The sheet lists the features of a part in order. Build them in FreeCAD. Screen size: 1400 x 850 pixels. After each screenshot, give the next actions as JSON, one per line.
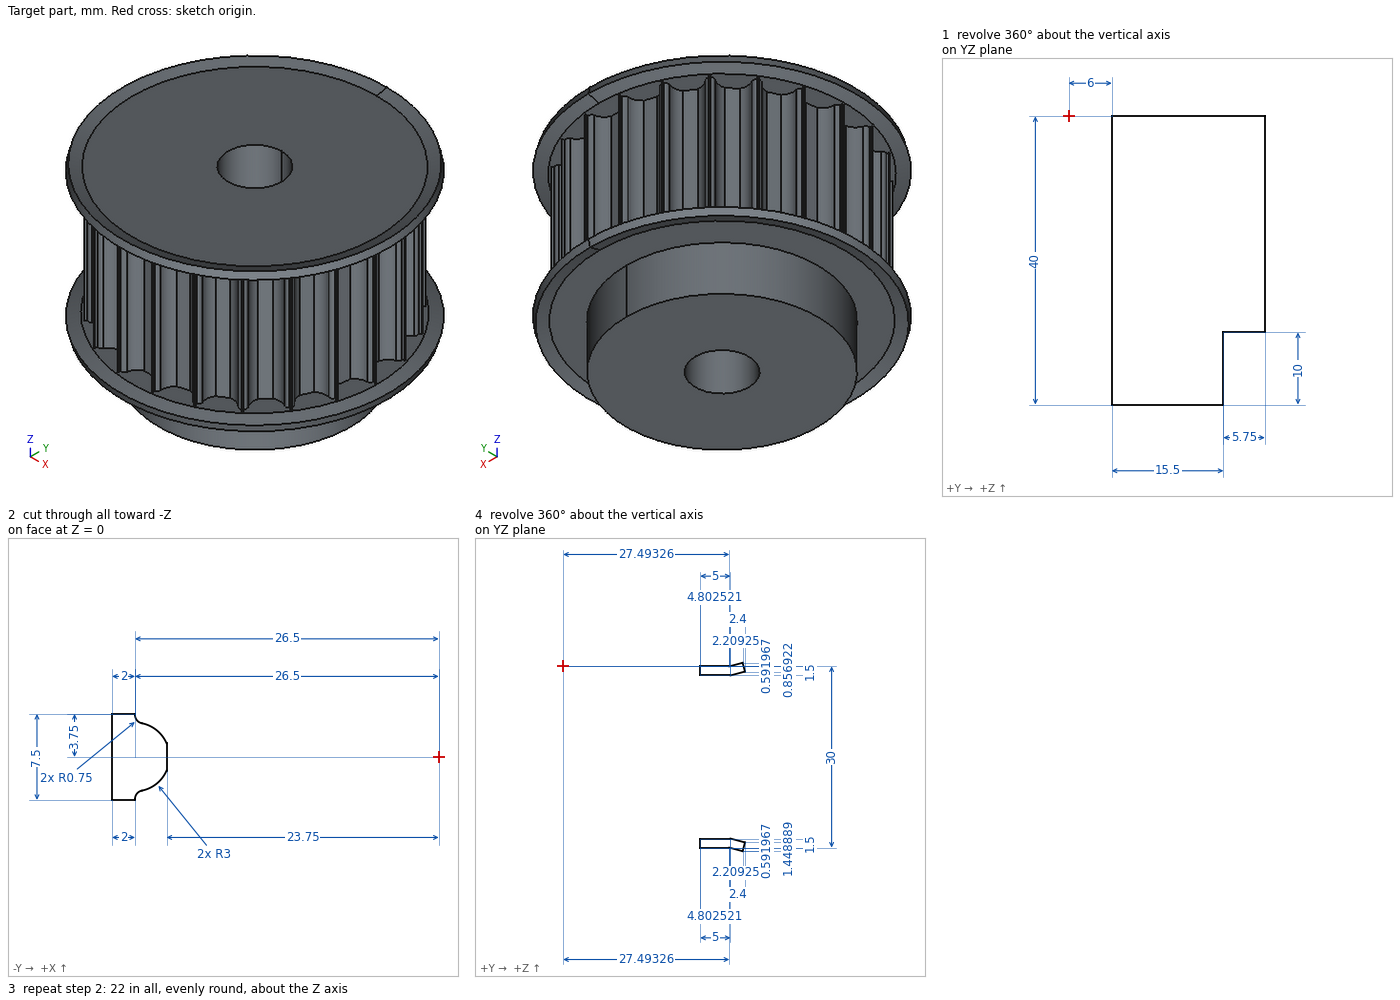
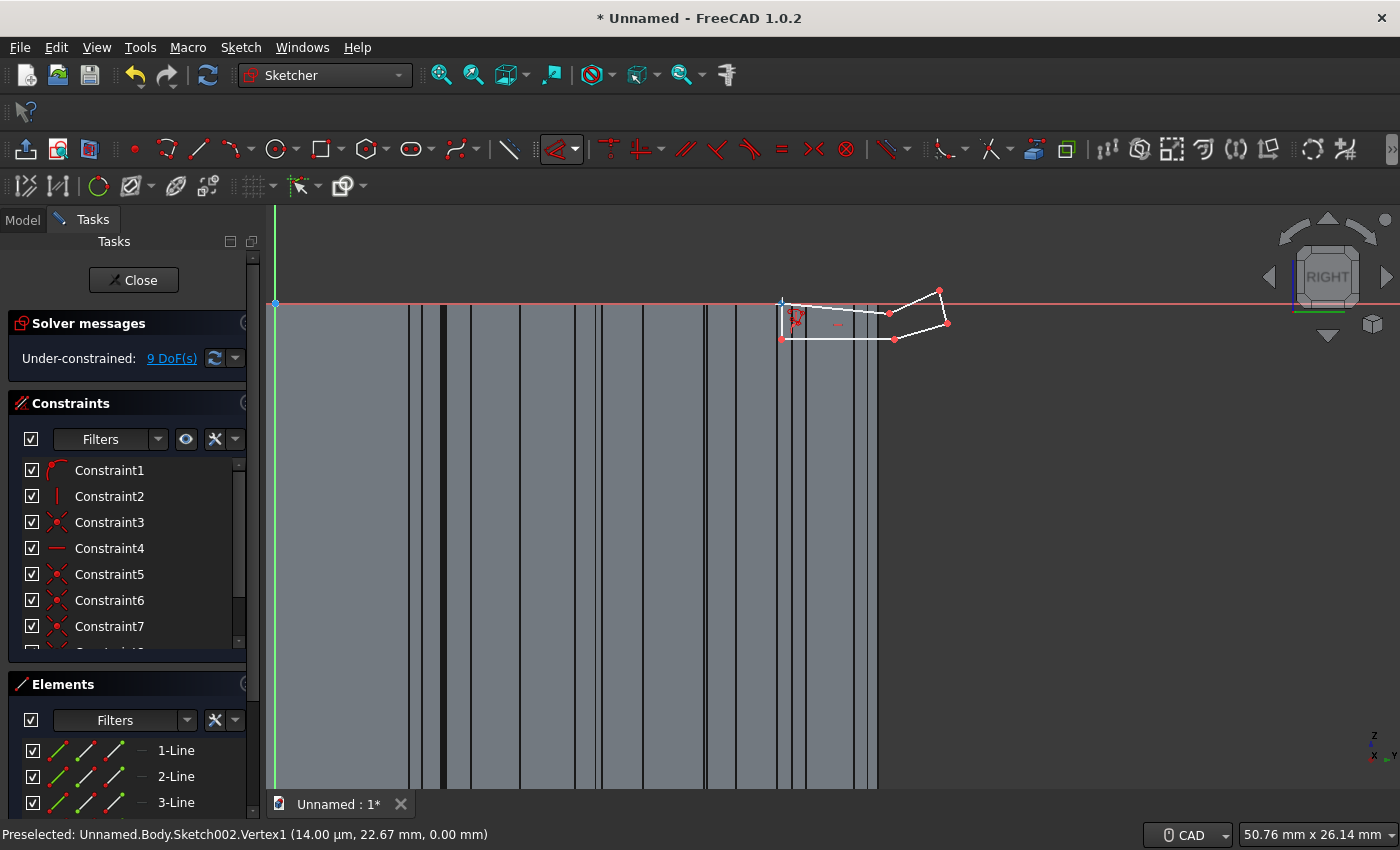
{"action": "scroll", "coordinate": [951, 325], "scroll_direction": "down", "scroll_amount": 3}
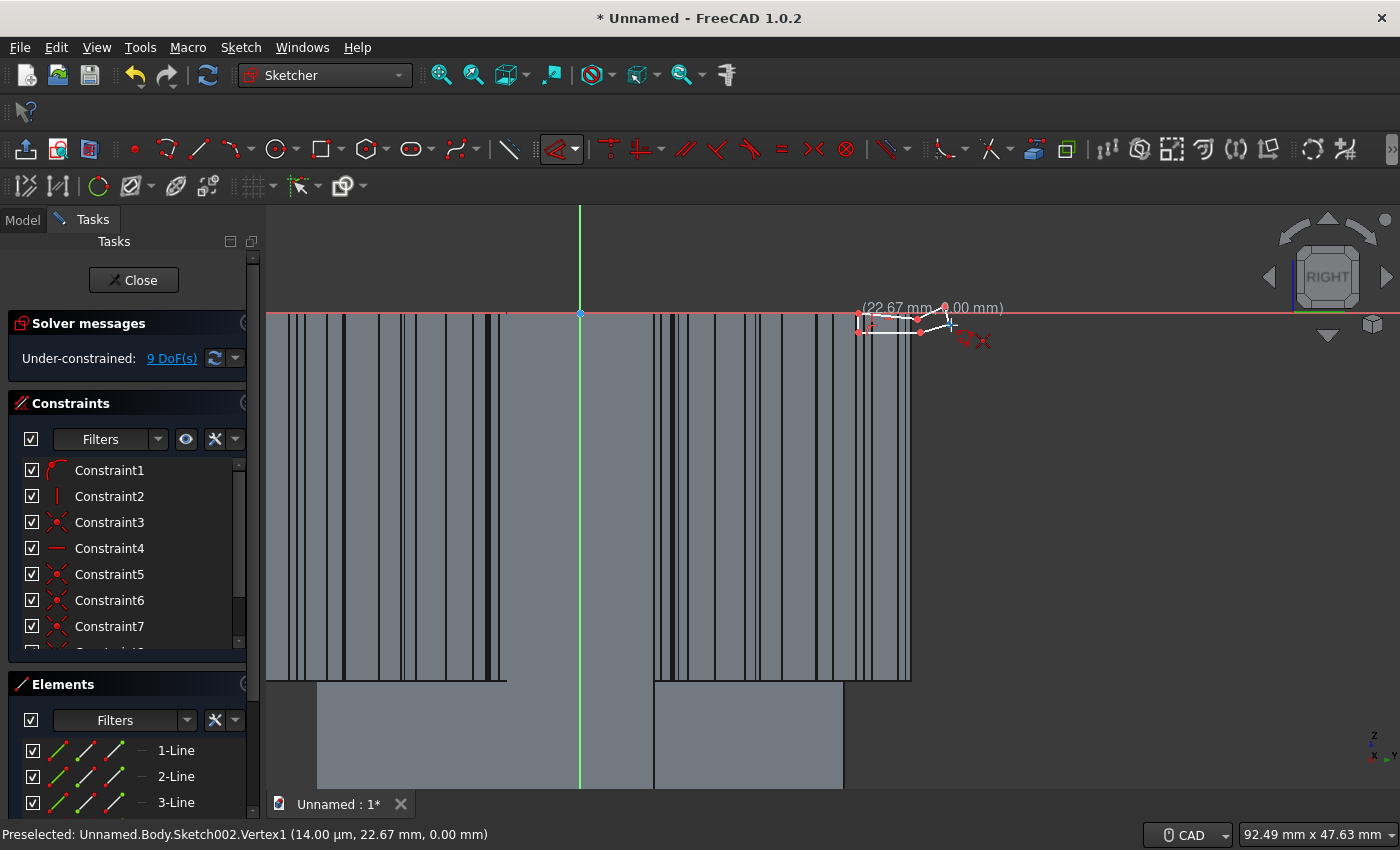
{"action": "left_click", "coordinate": [859, 663]}
{"action": "left_click", "coordinate": [859, 681]}
{"action": "left_click", "coordinate": [917, 681]}
{"action": "left_click", "coordinate": [945, 688]}
{"action": "left_click", "coordinate": [949, 671]}
{"action": "left_click", "coordinate": [920, 663]}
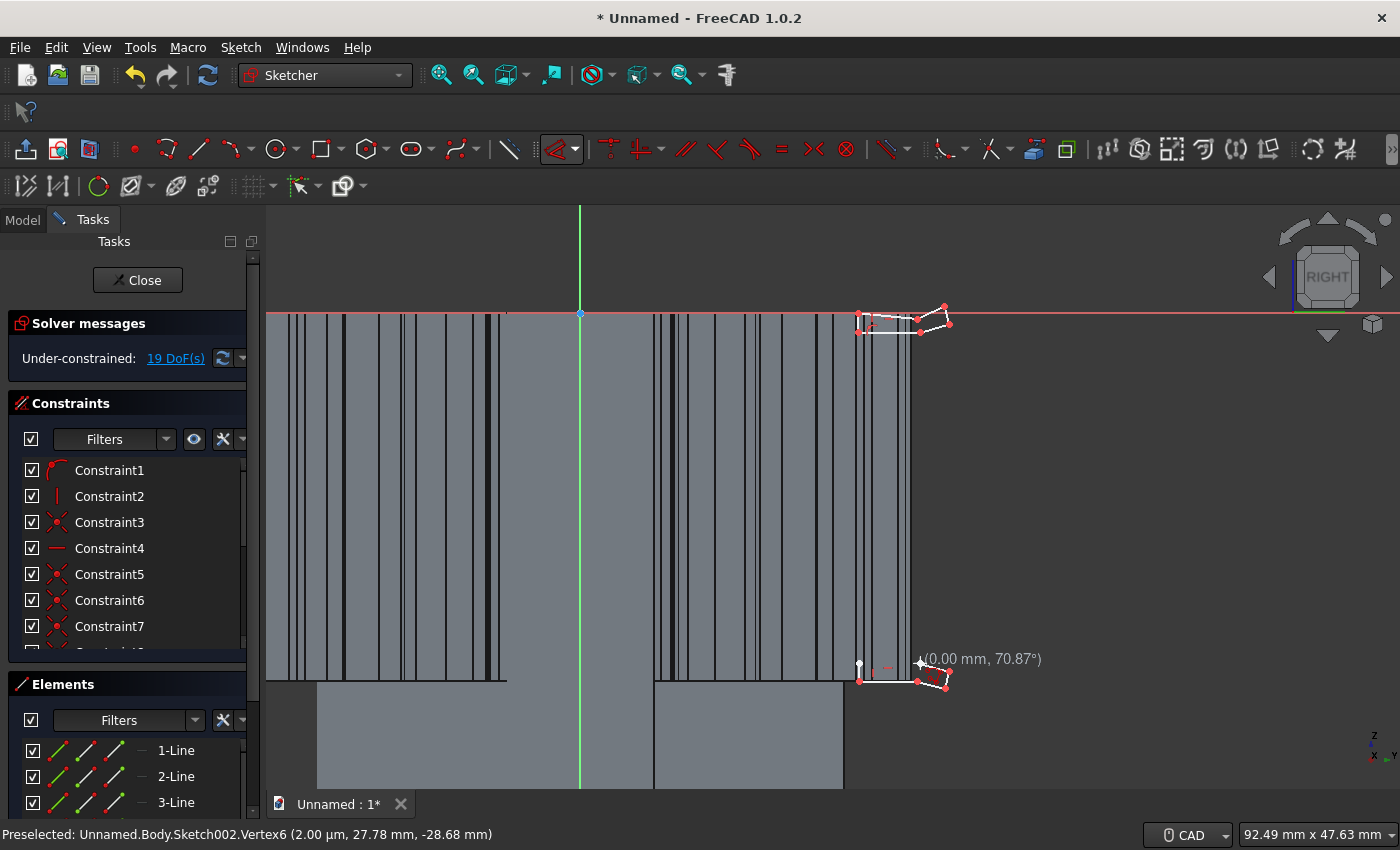
{"action": "scroll", "coordinate": [859, 663], "scroll_direction": "up", "scroll_amount": 3}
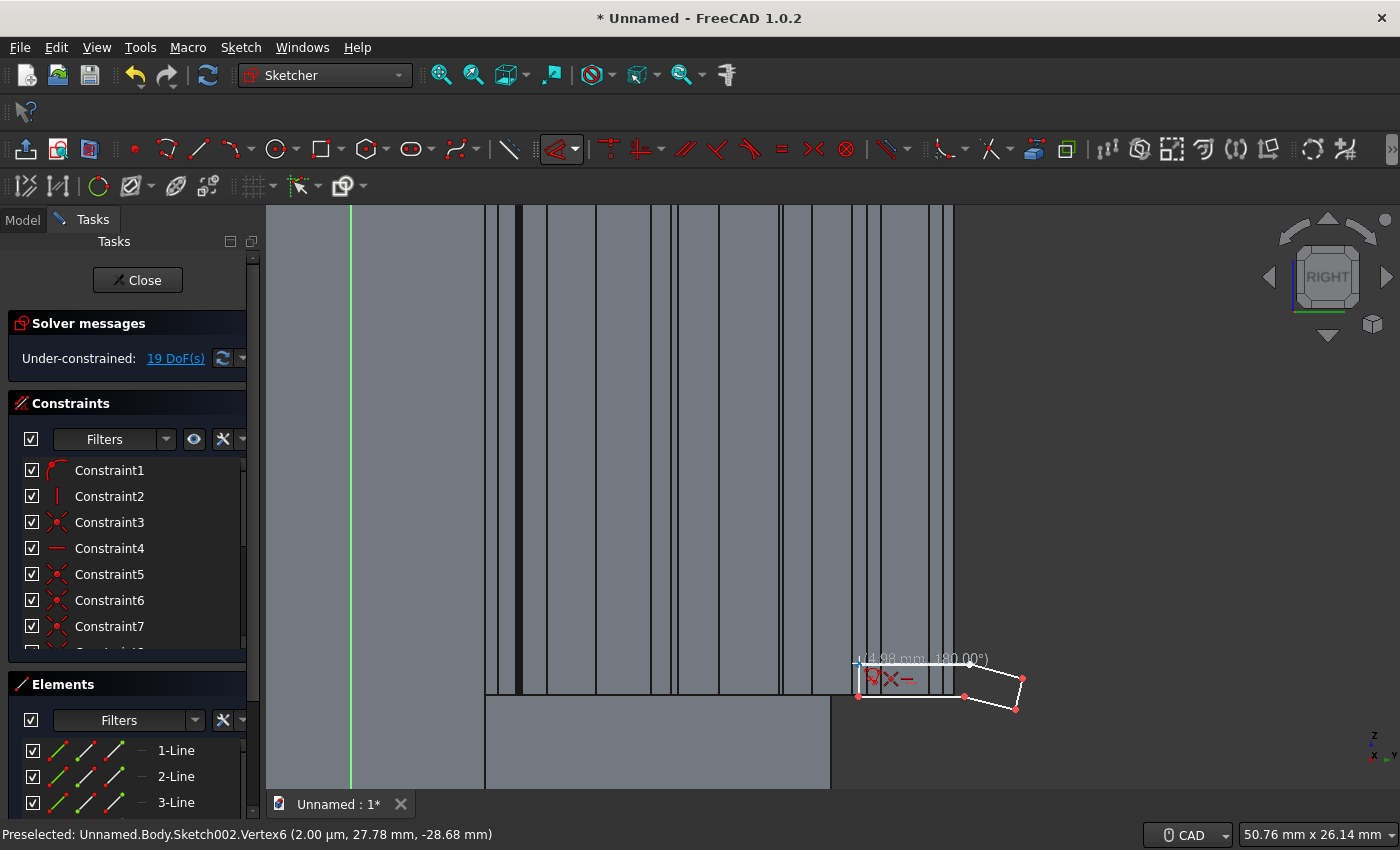
{"action": "left_click", "coordinate": [859, 664]}
{"action": "key", "text": "Escape"}
{"action": "key", "text": "Escape"}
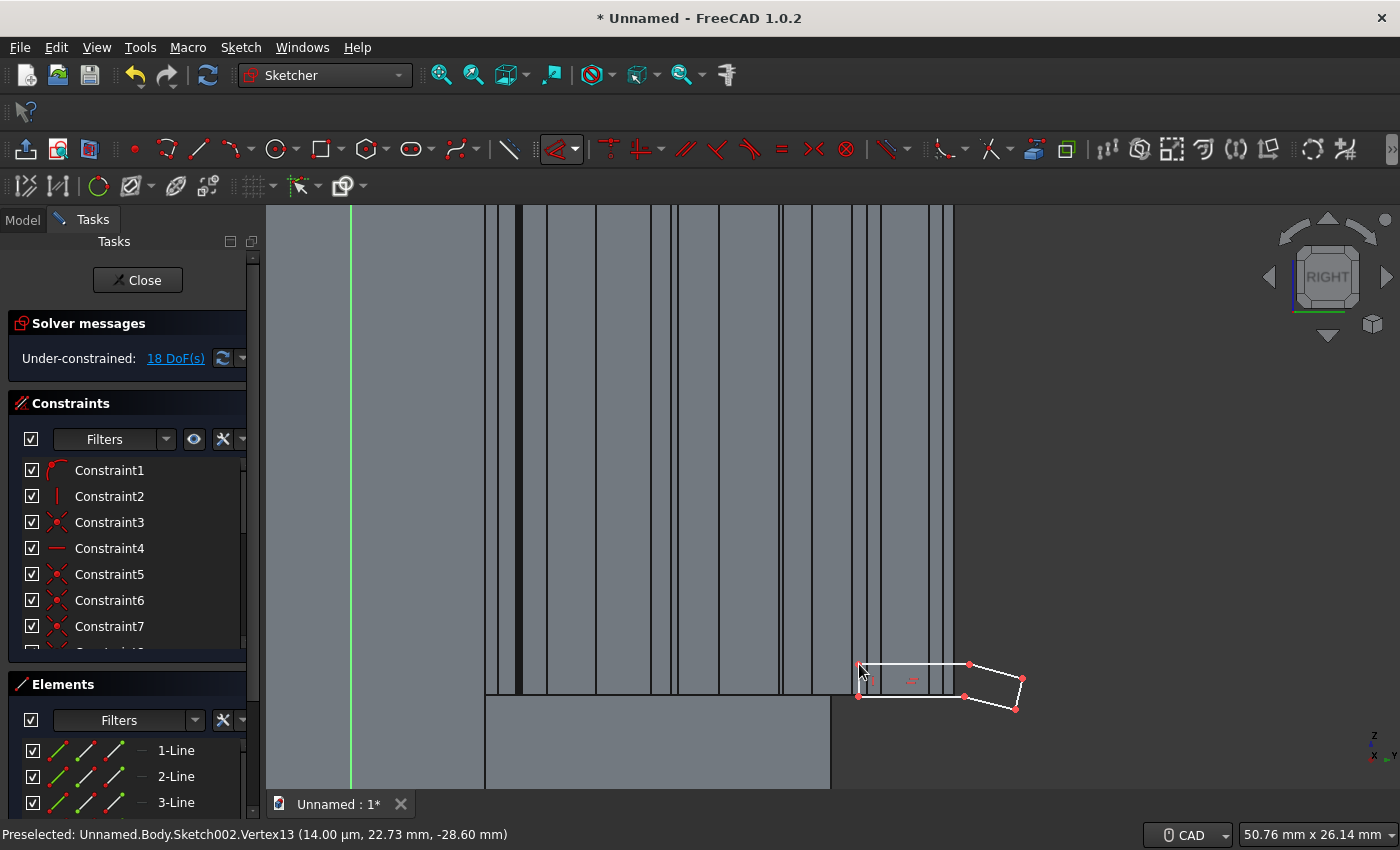
{"action": "scroll", "coordinate": [859, 663], "scroll_direction": "down", "scroll_amount": 3}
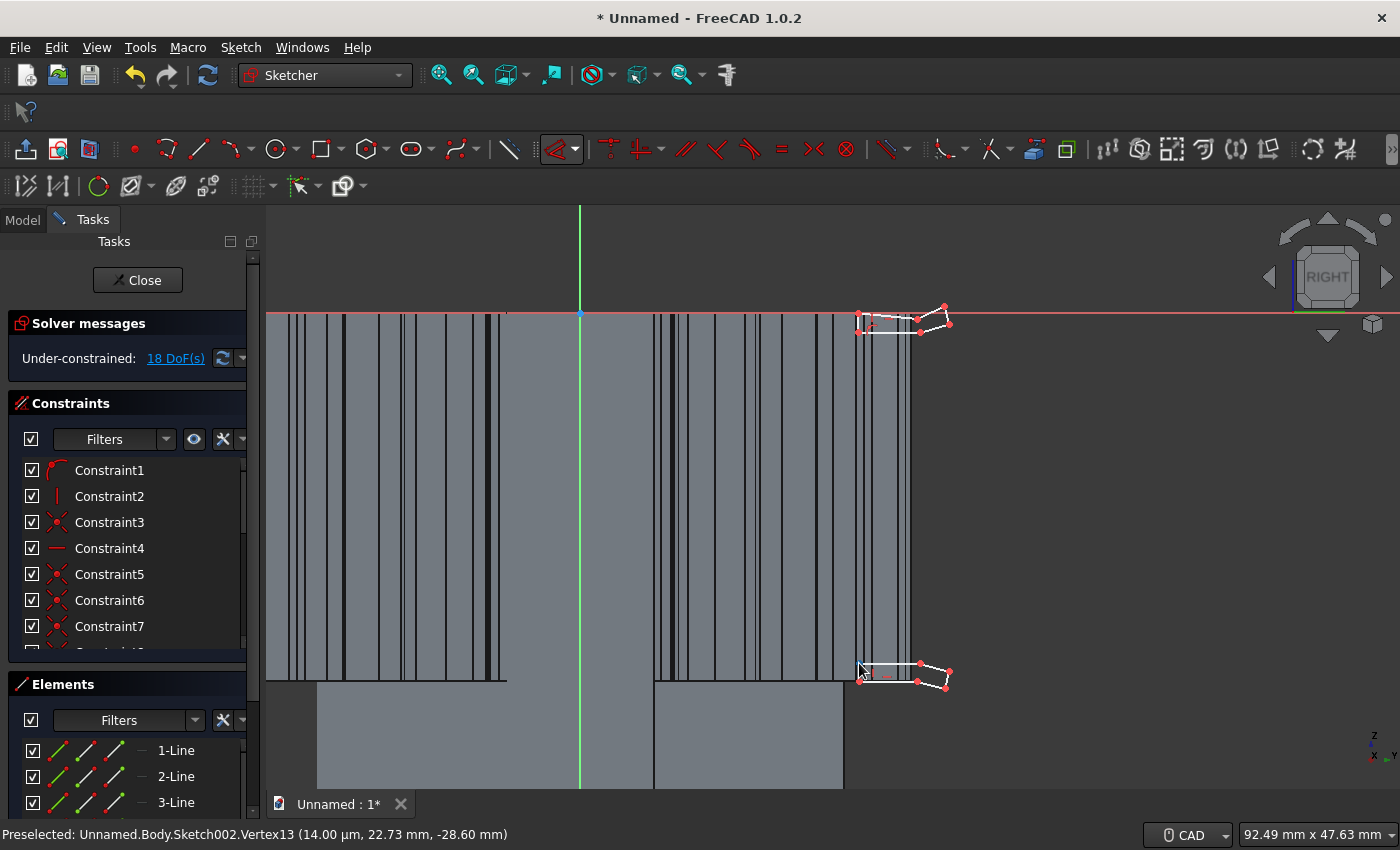
{"action": "left_click", "coordinate": [905, 318]}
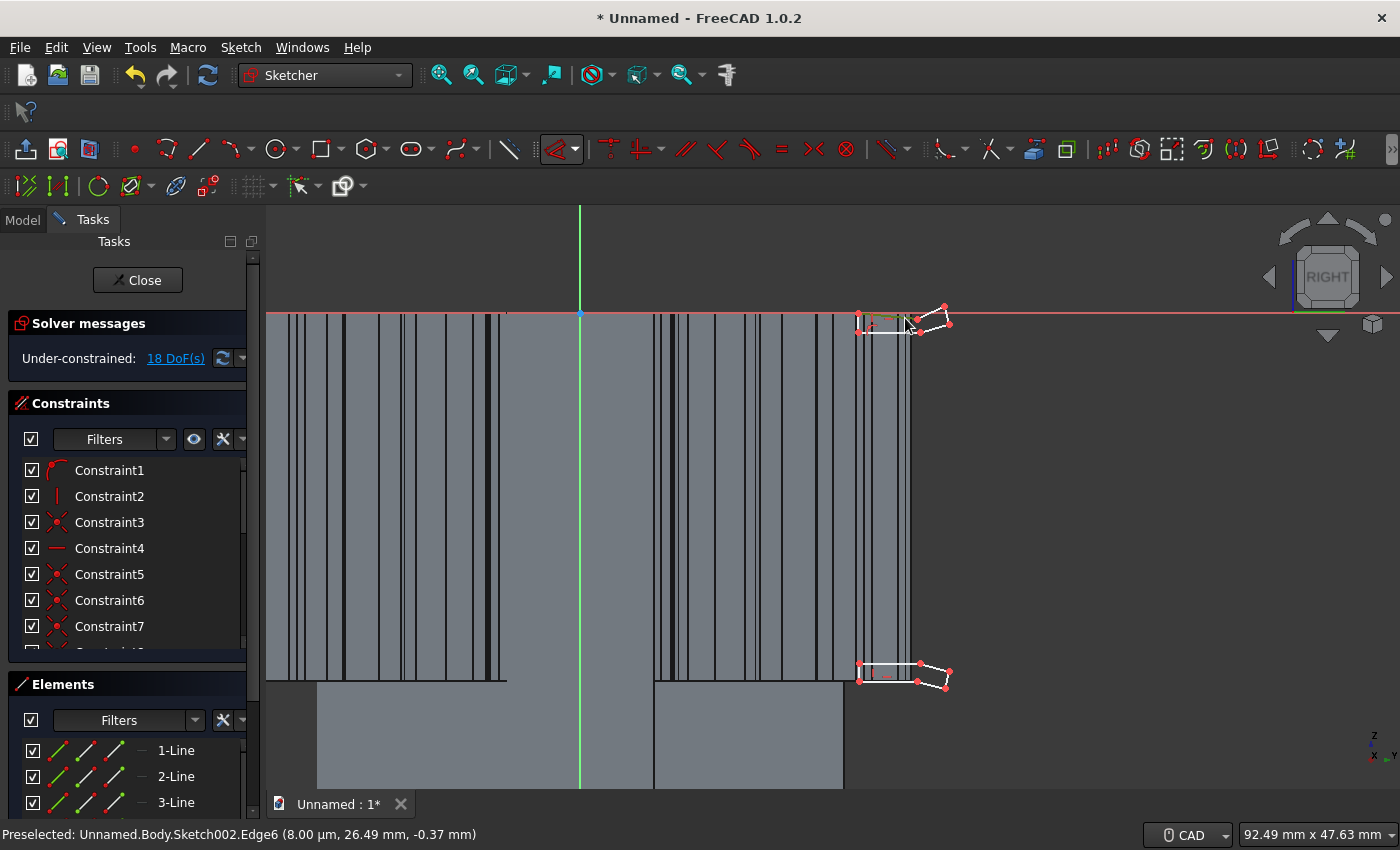
{"action": "key", "text": "h"}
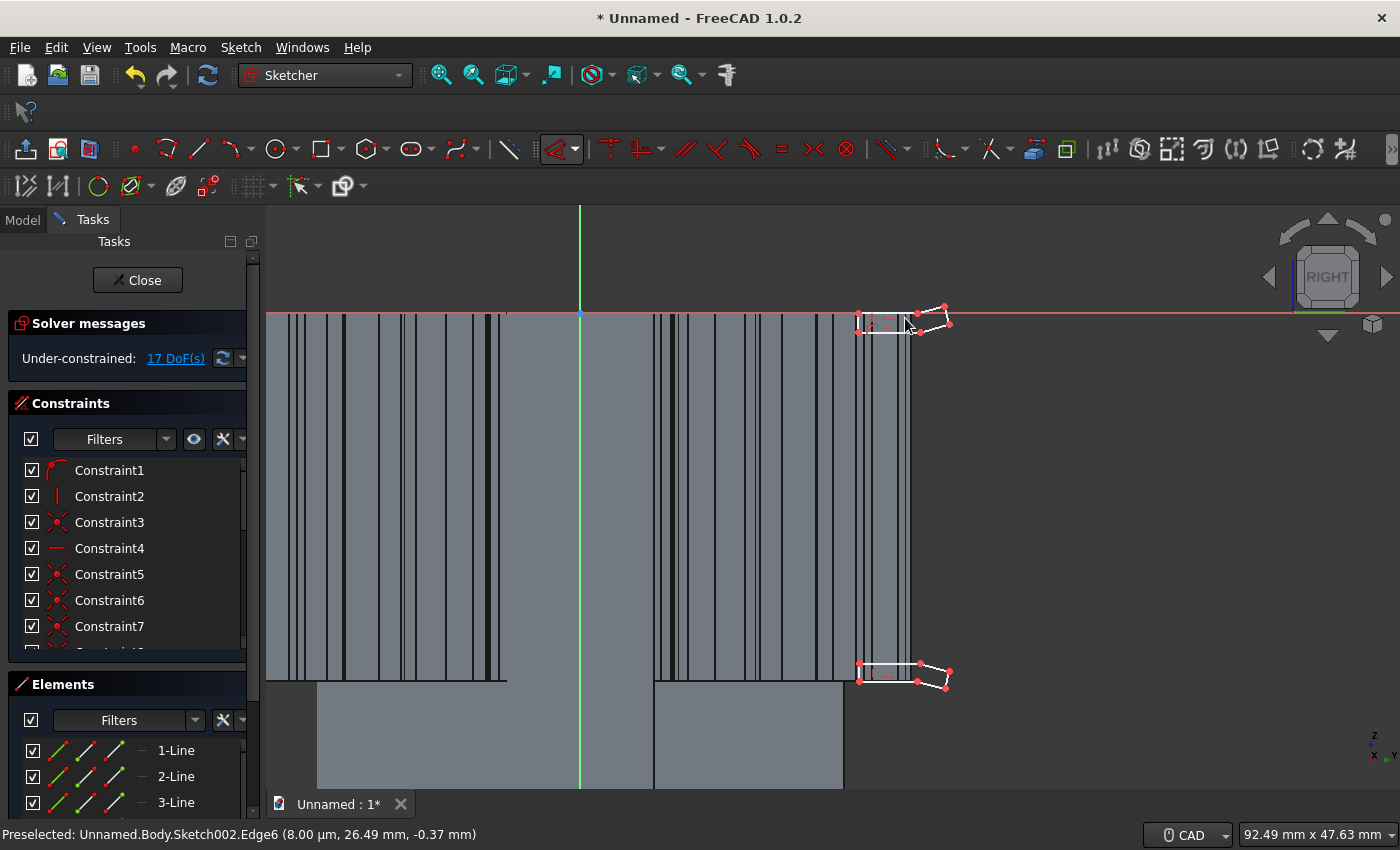
{"action": "left_click", "coordinate": [902, 333]}